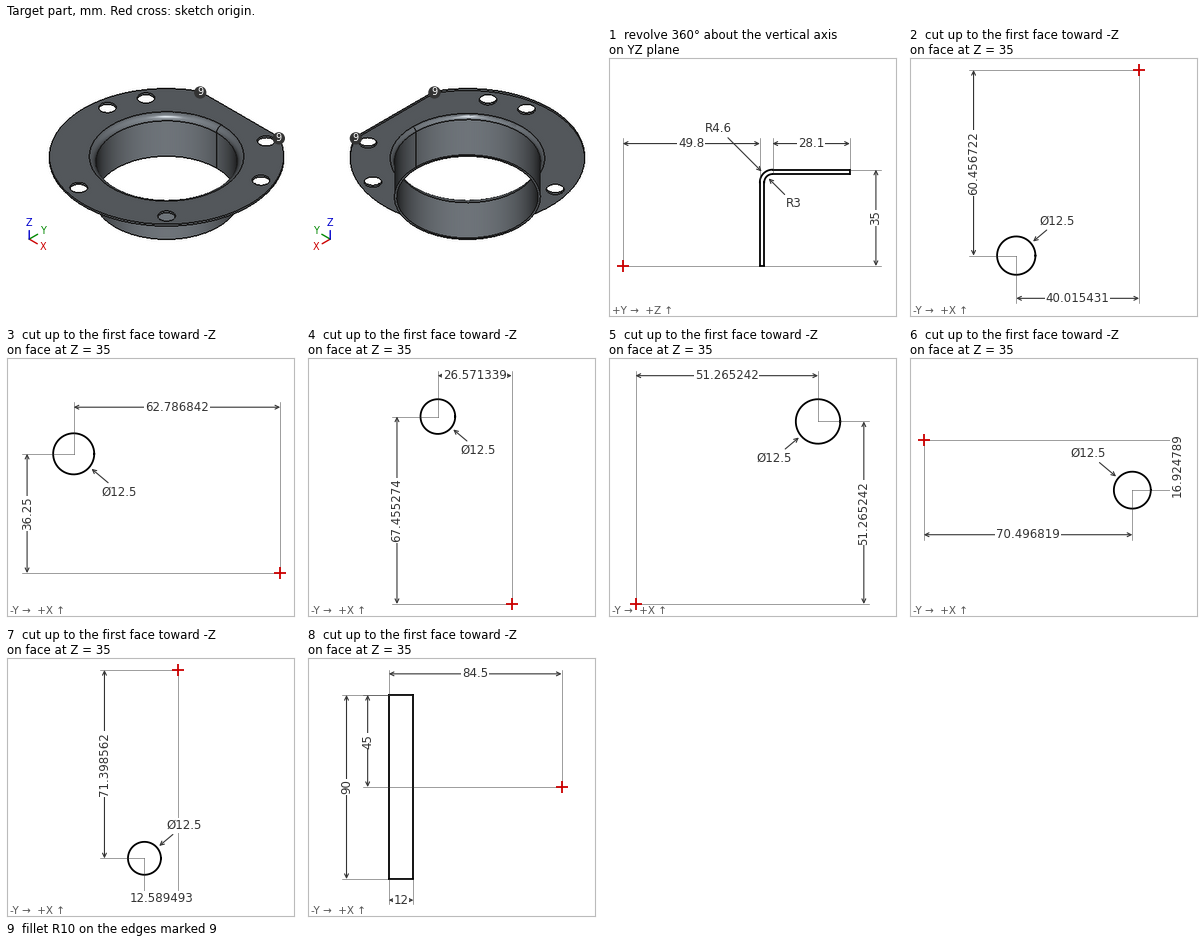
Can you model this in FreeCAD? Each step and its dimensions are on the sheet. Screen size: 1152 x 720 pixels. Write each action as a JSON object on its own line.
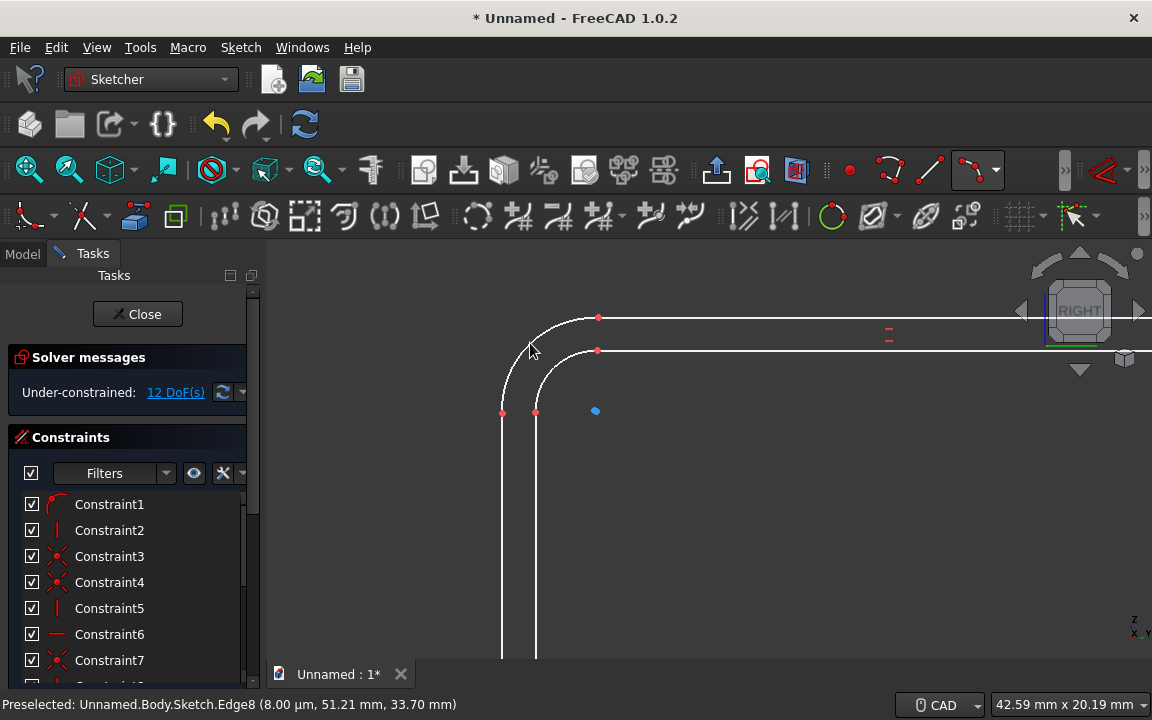
{"action": "left_click", "coordinate": [502, 602]}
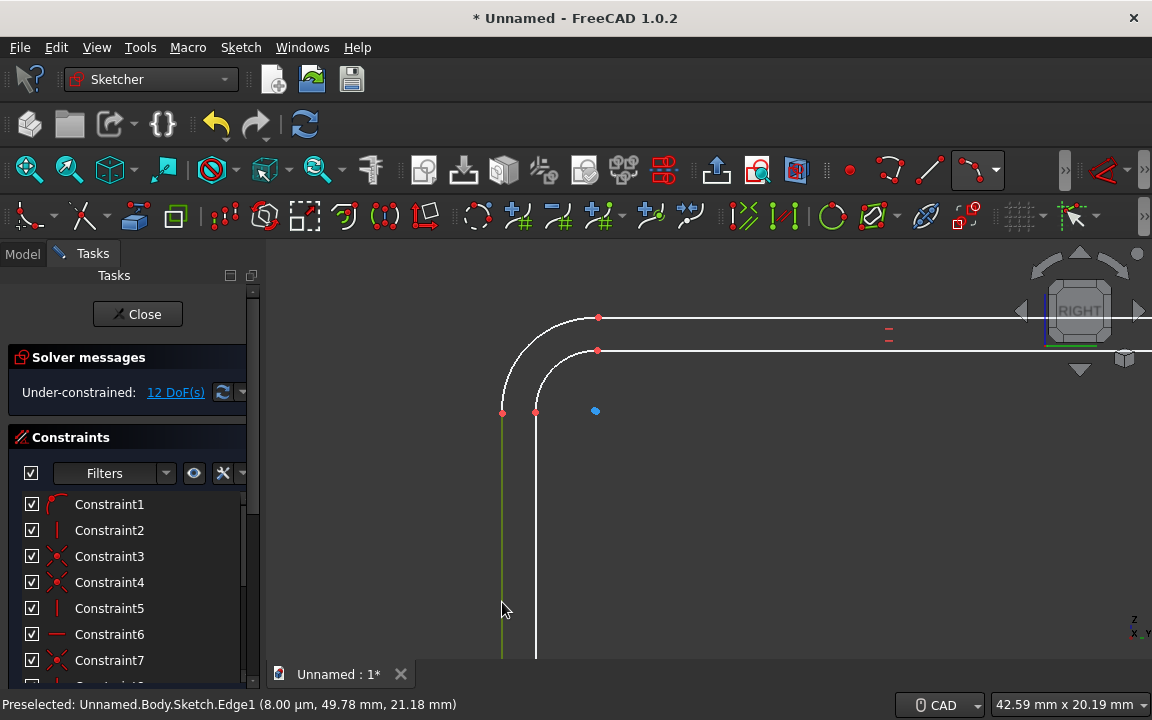
{"action": "left_click", "coordinate": [554, 327]}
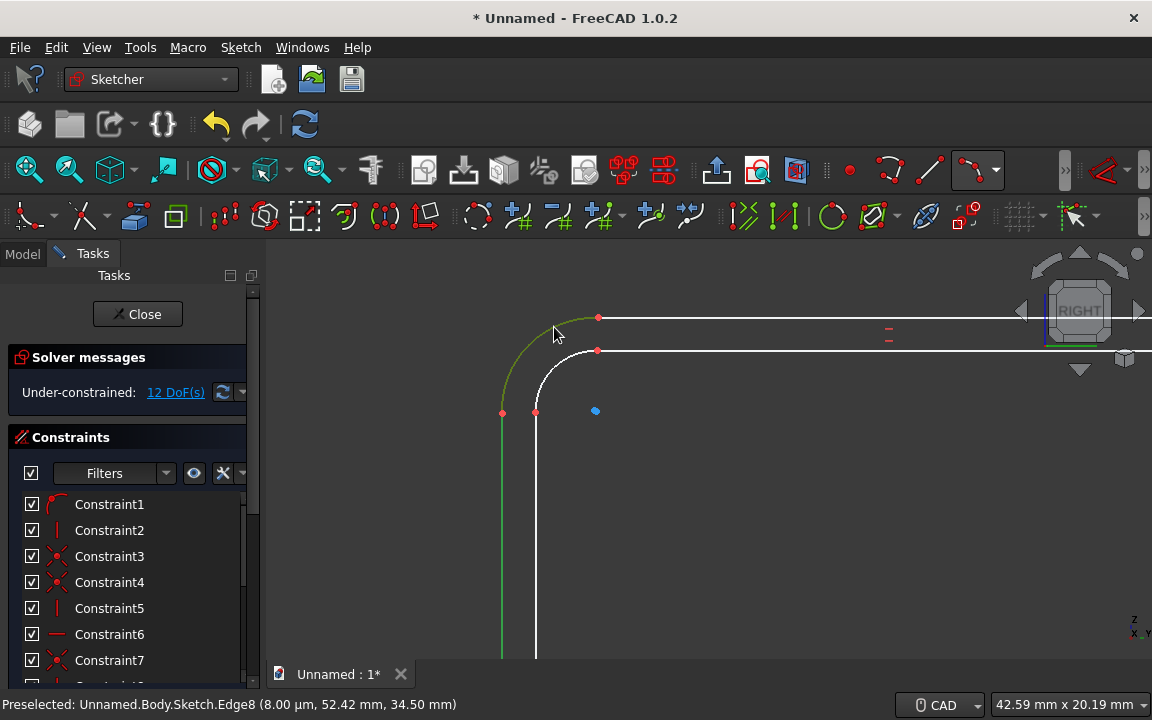
{"action": "key", "text": "t"}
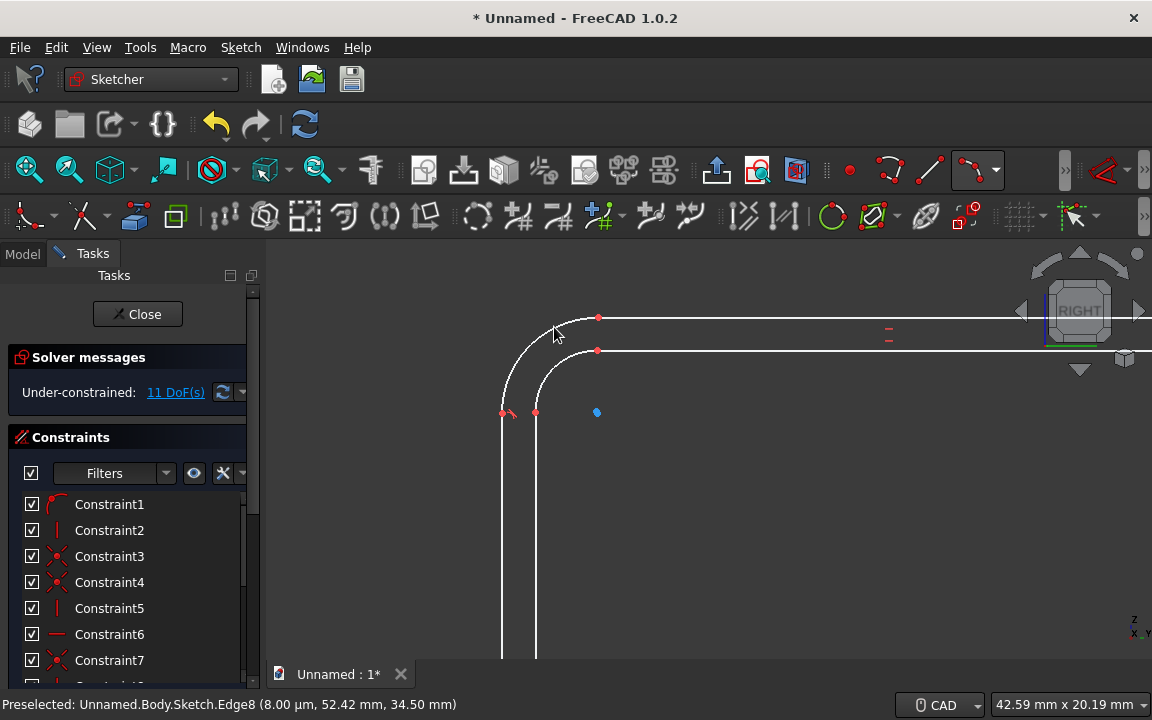
{"action": "left_click", "coordinate": [536, 597]}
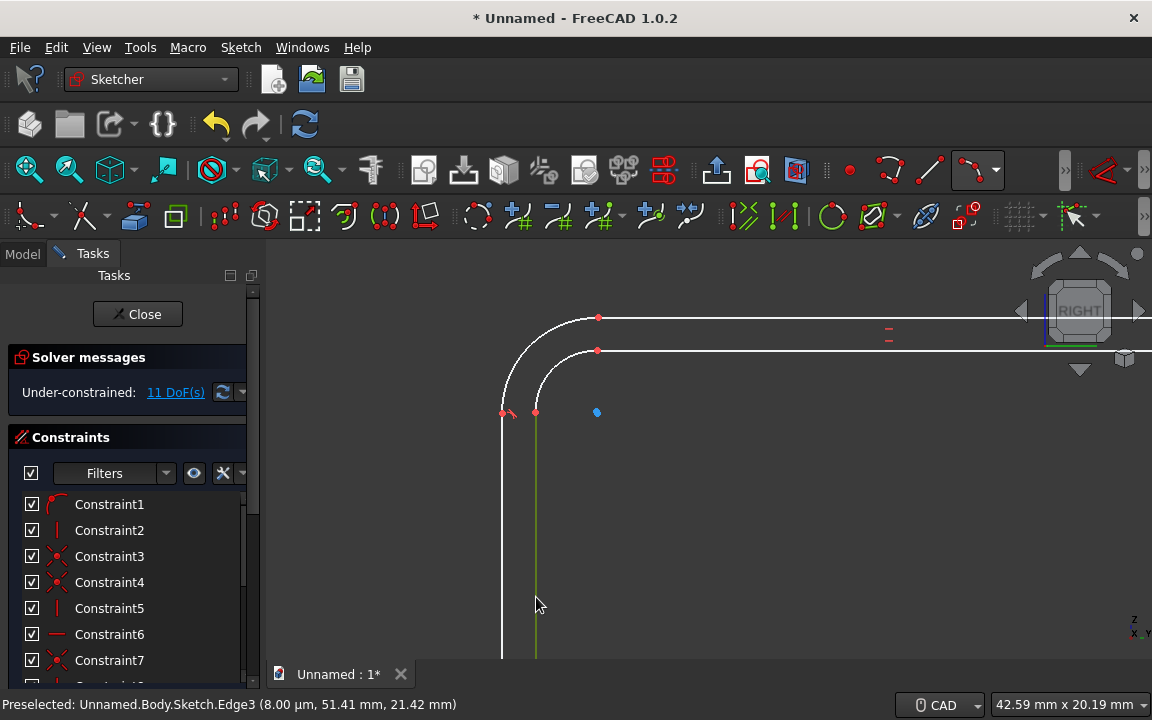
{"action": "left_click", "coordinate": [569, 357]}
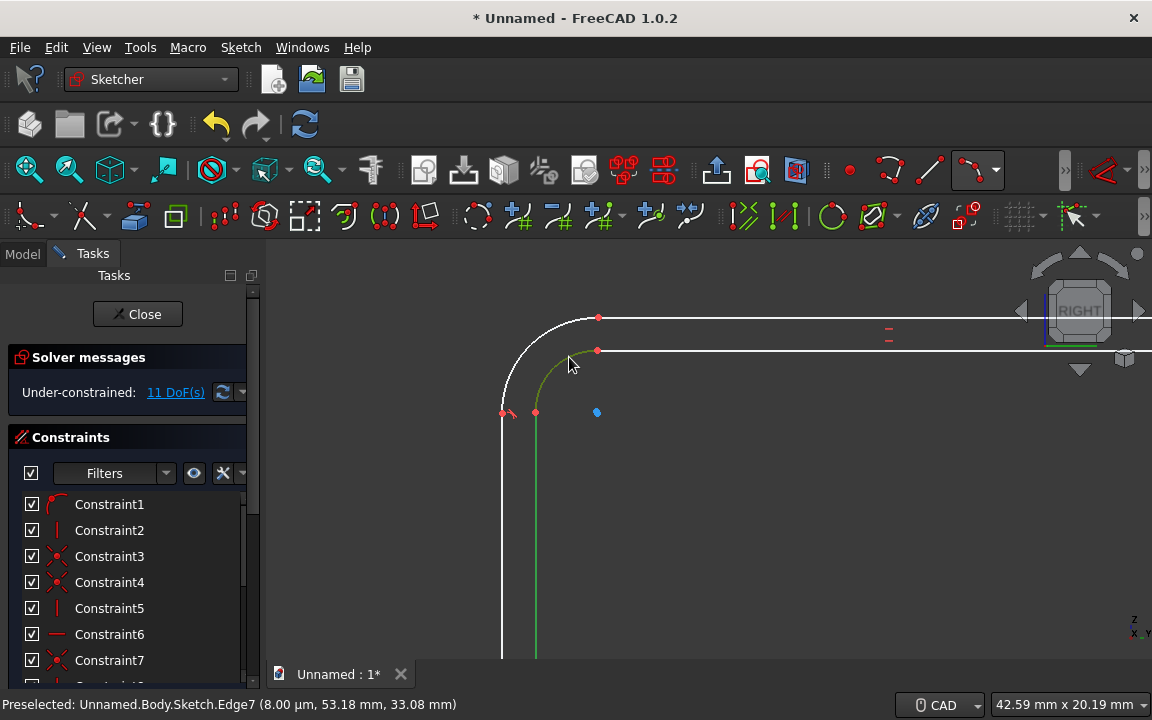
{"action": "key", "text": "t"}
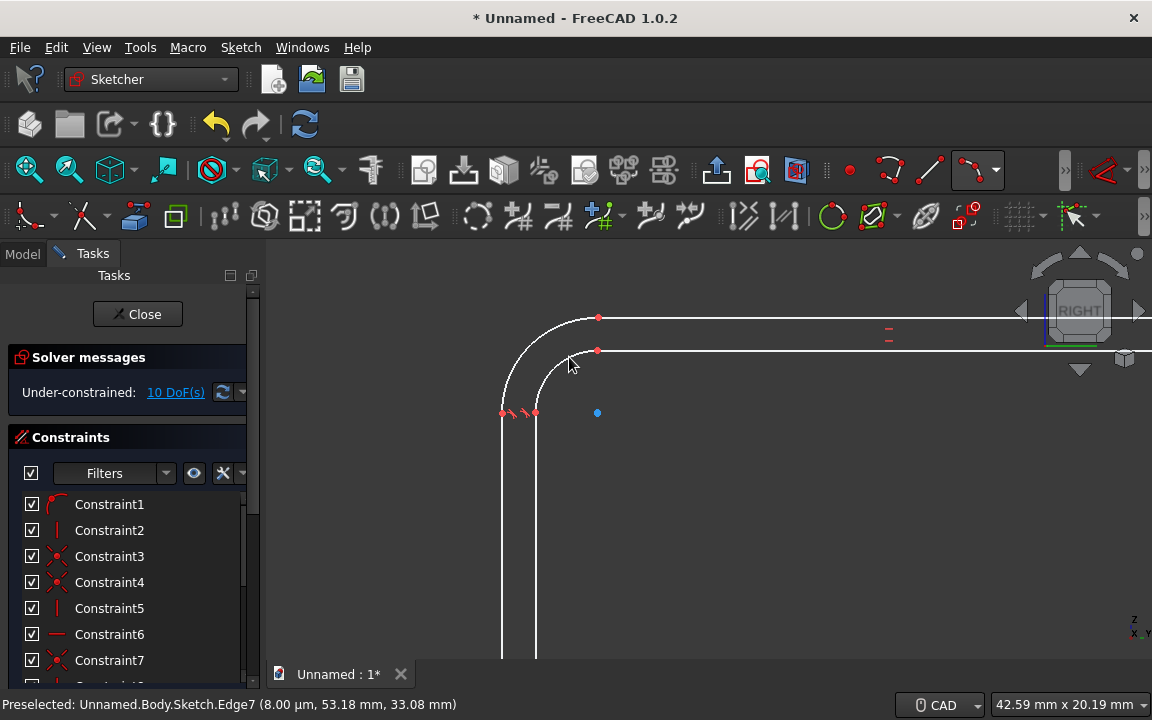
{"action": "left_click", "coordinate": [773, 351]}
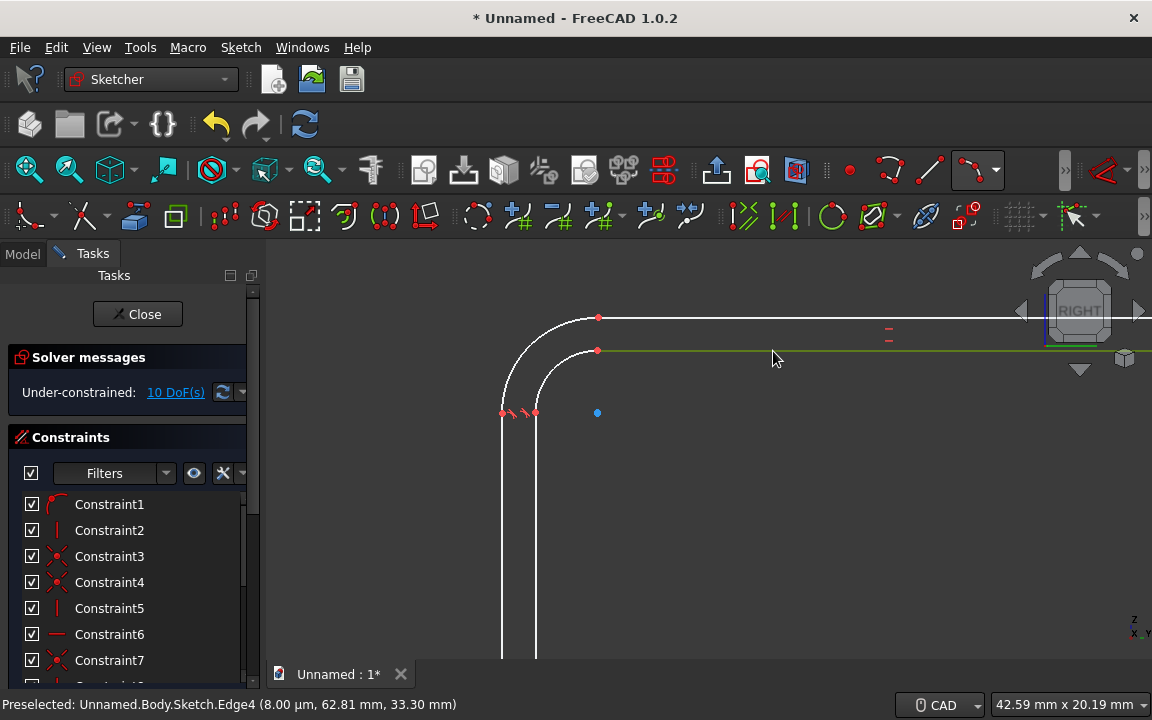
{"action": "left_click", "coordinate": [569, 357]}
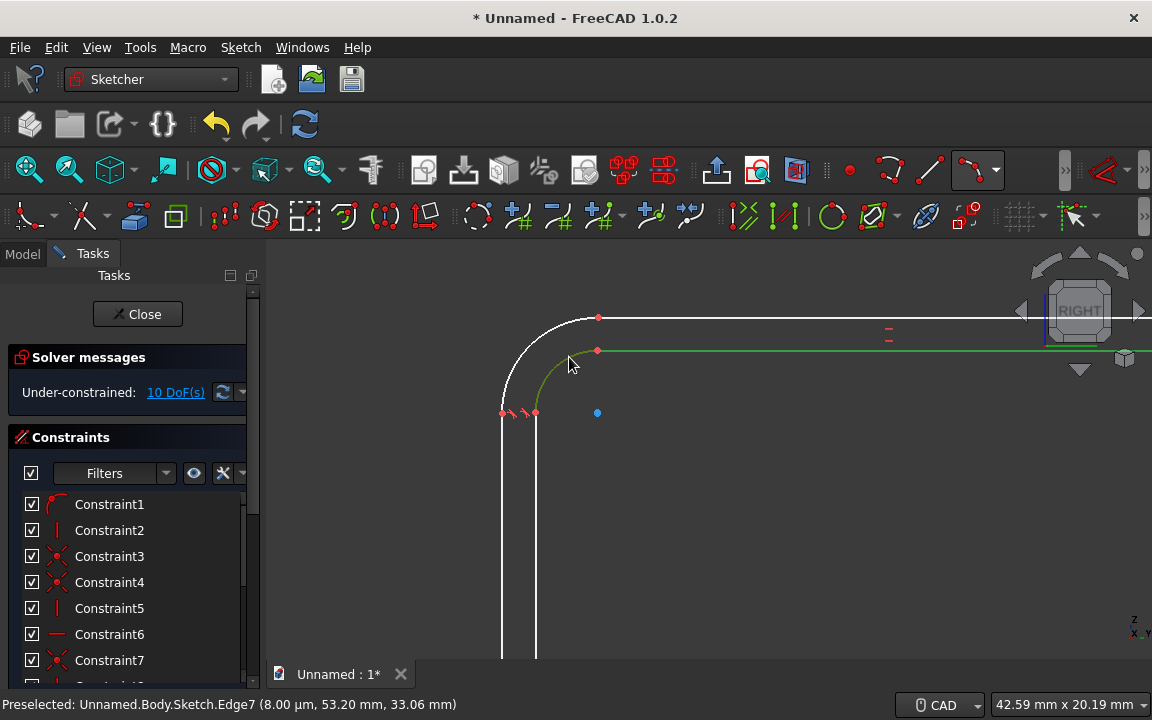
{"action": "key", "text": "t"}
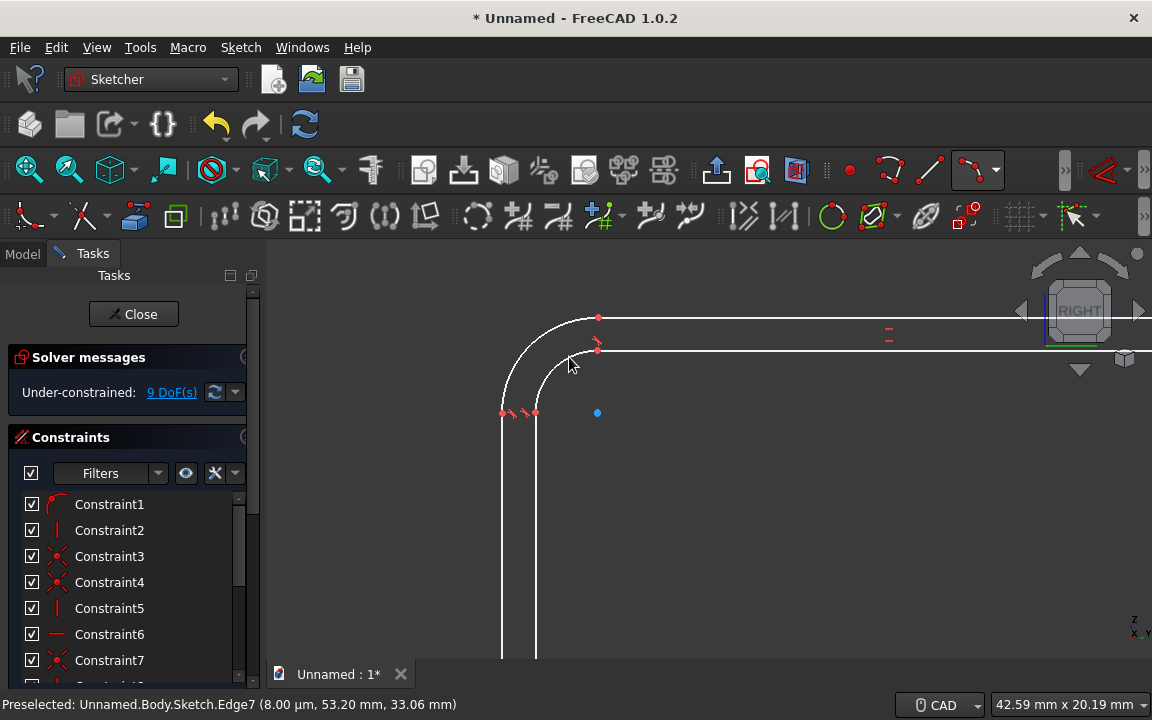
{"action": "left_click", "coordinate": [773, 318]}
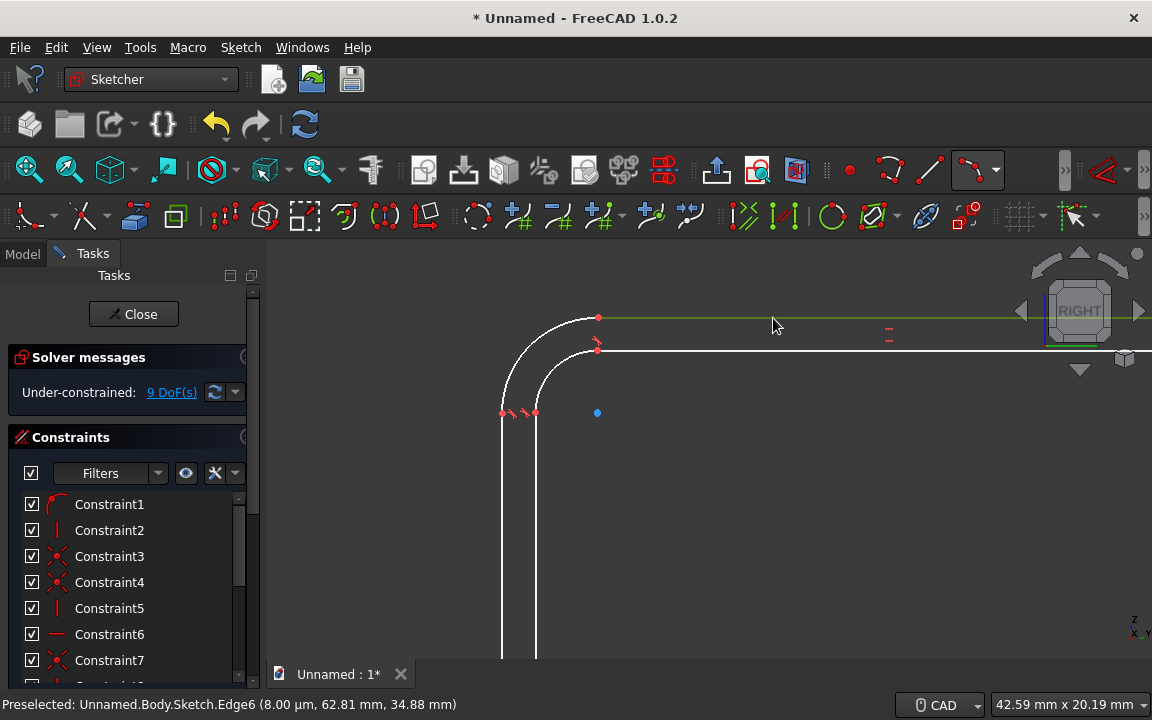
{"action": "left_click", "coordinate": [555, 328]}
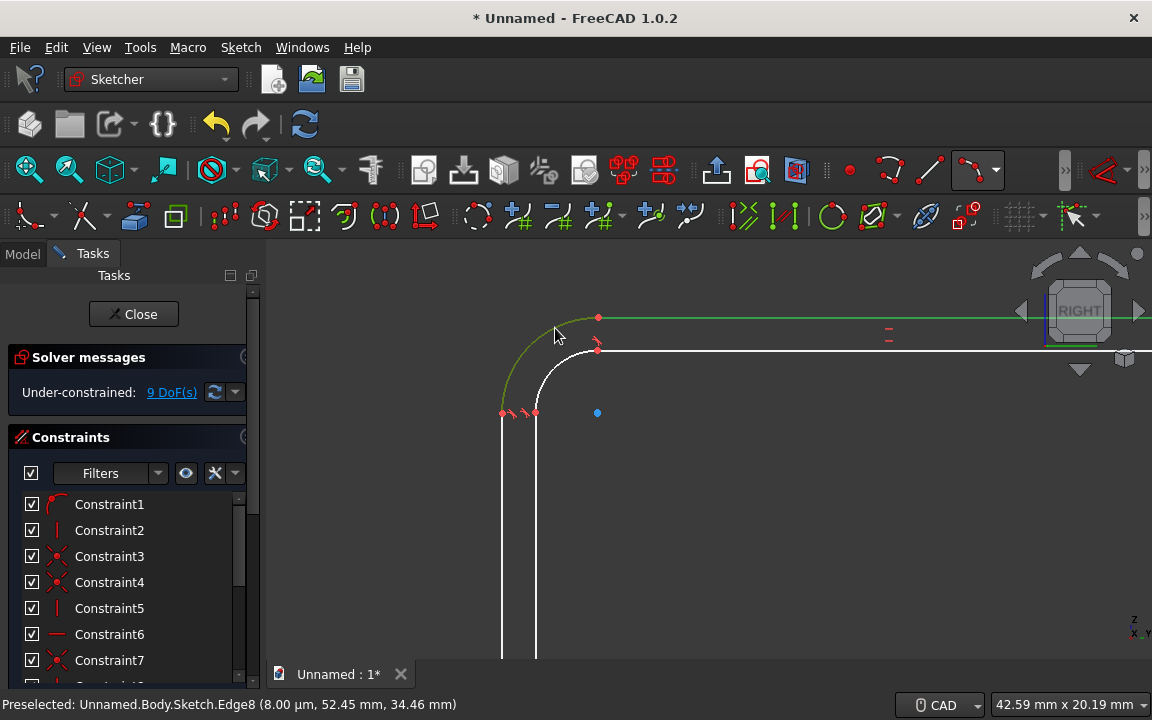
{"action": "key", "text": "t"}